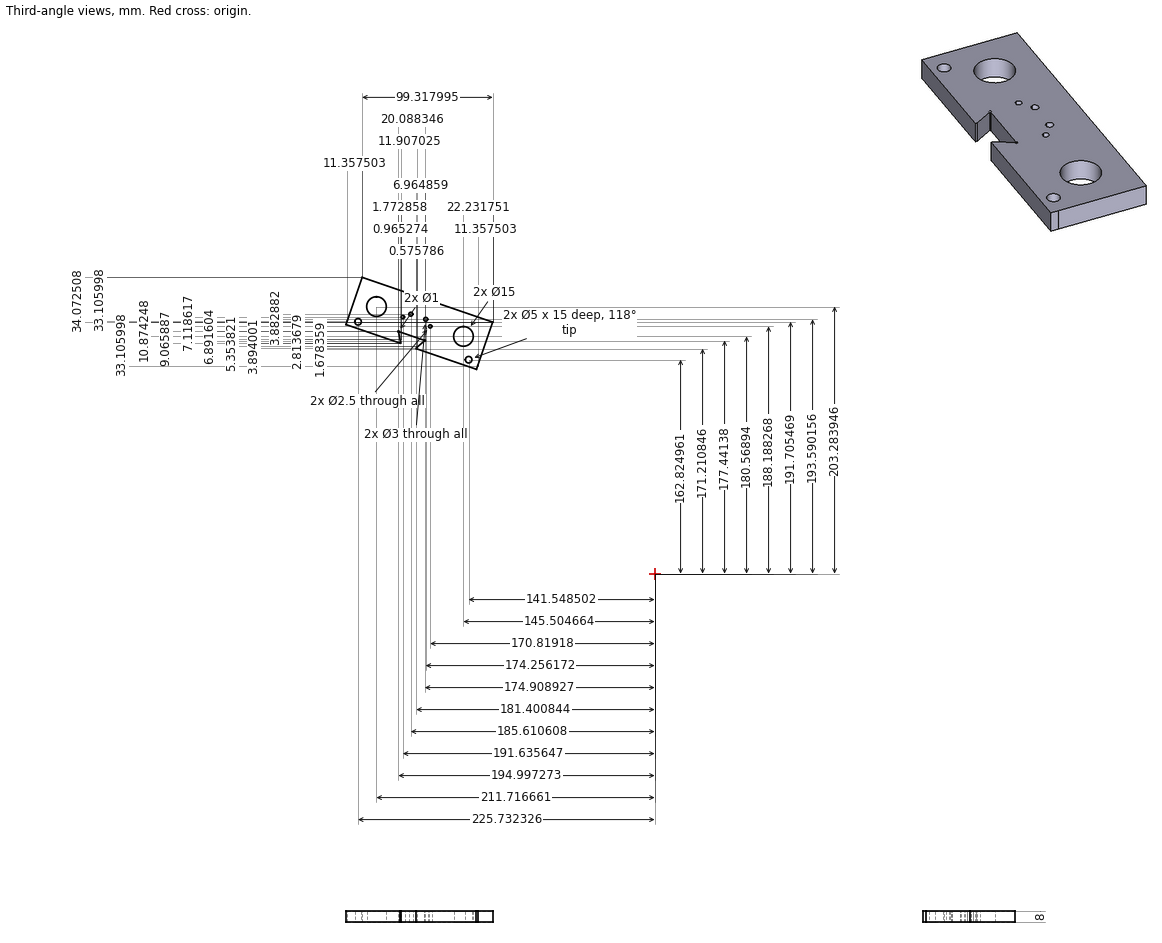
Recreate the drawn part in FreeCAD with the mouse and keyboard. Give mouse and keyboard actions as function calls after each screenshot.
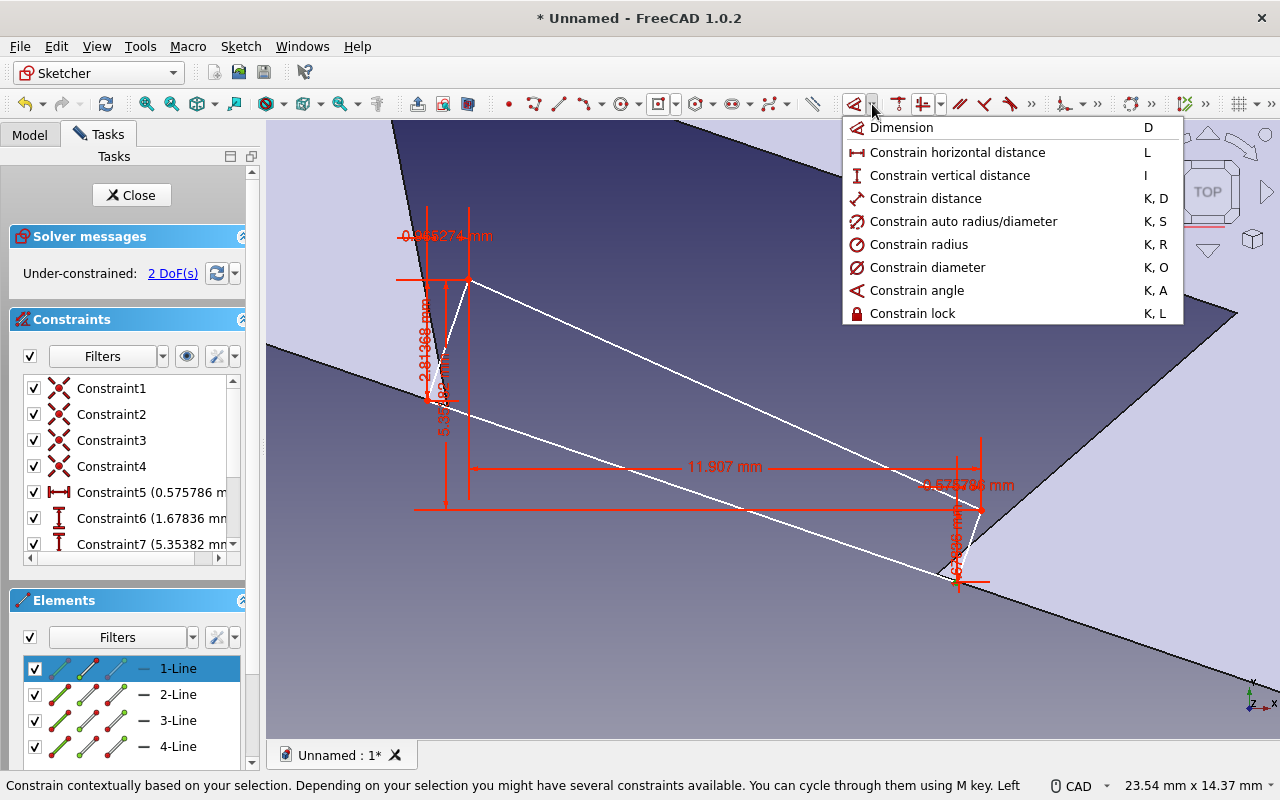
click(1013, 152)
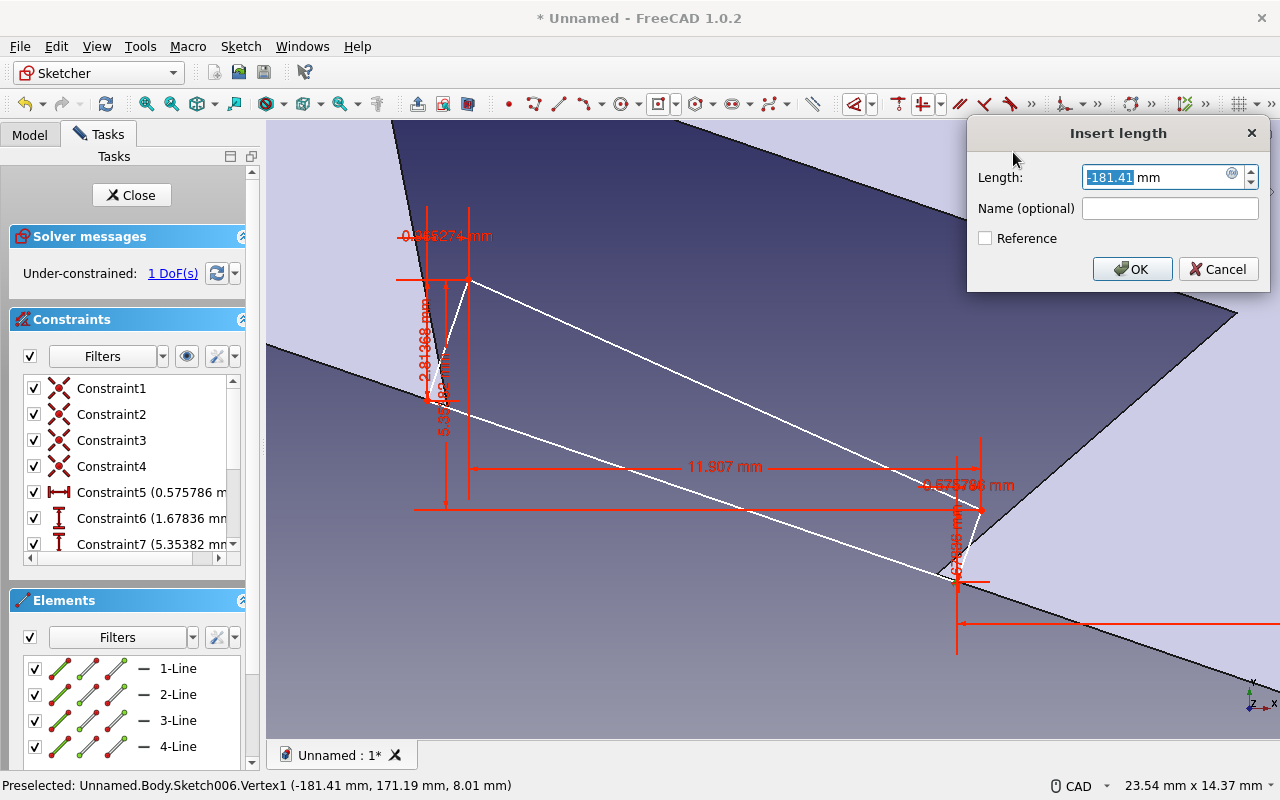
text(-181.400844)
key(Return)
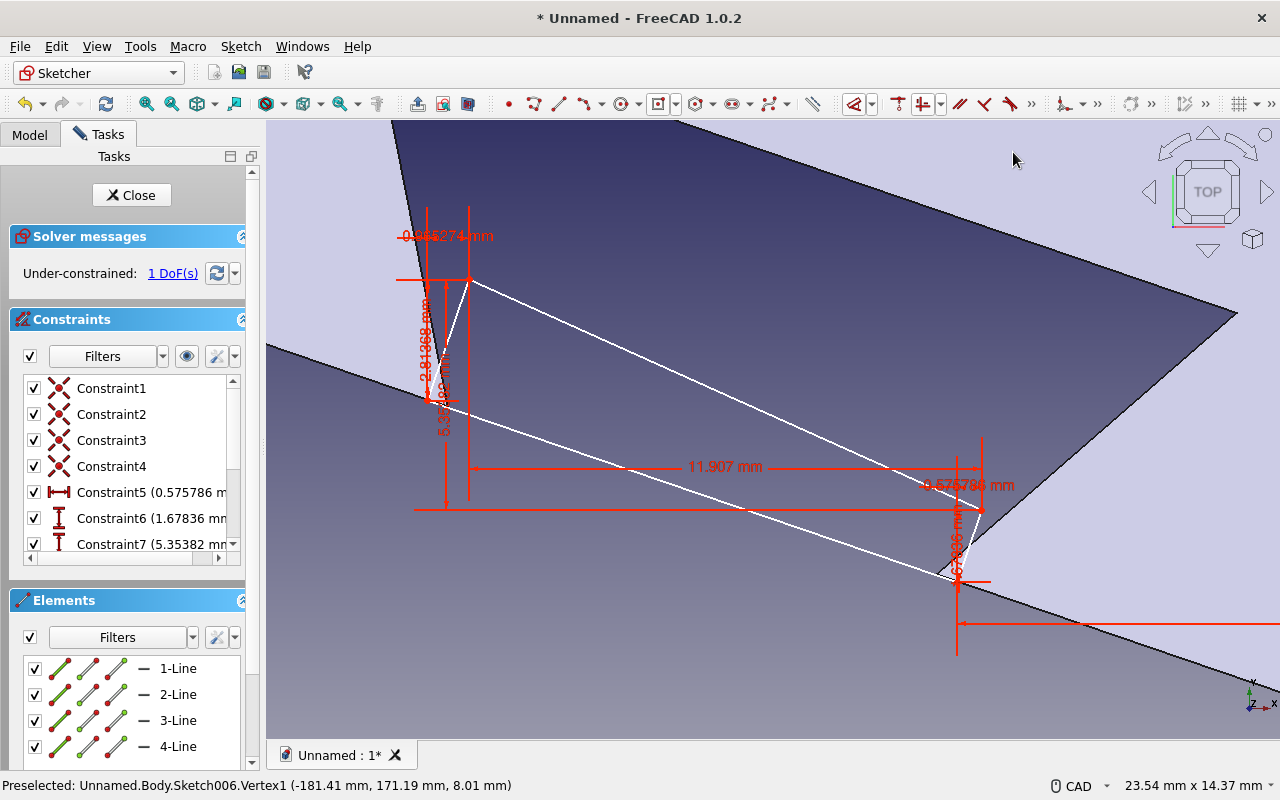
click(957, 582)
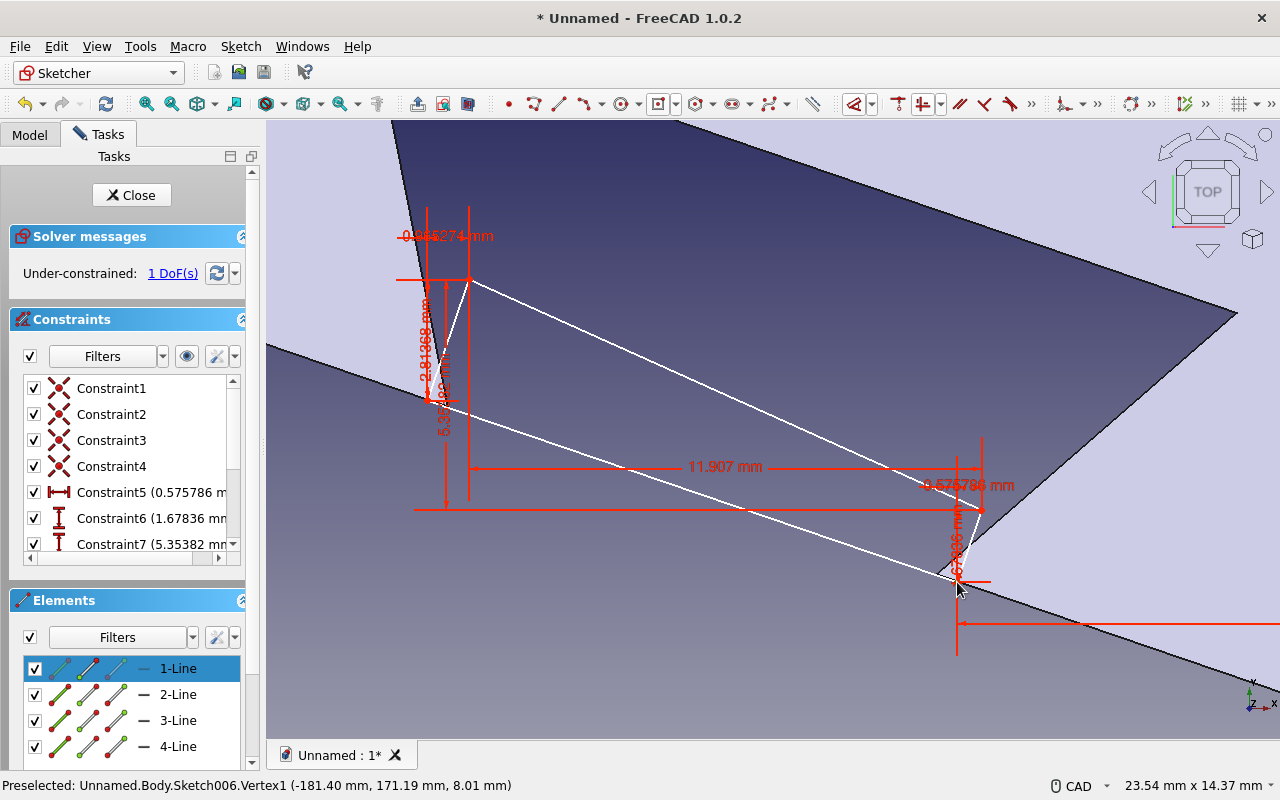
click(872, 104)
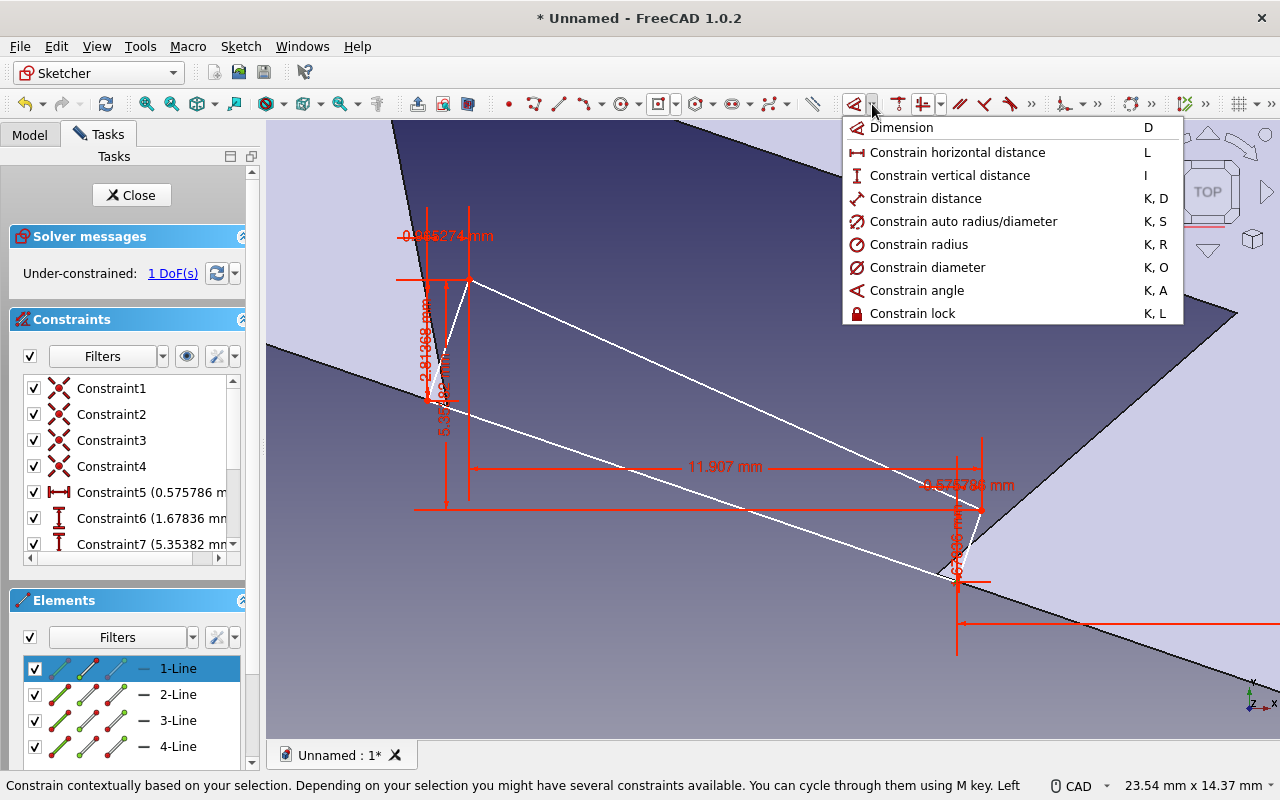
click(1013, 176)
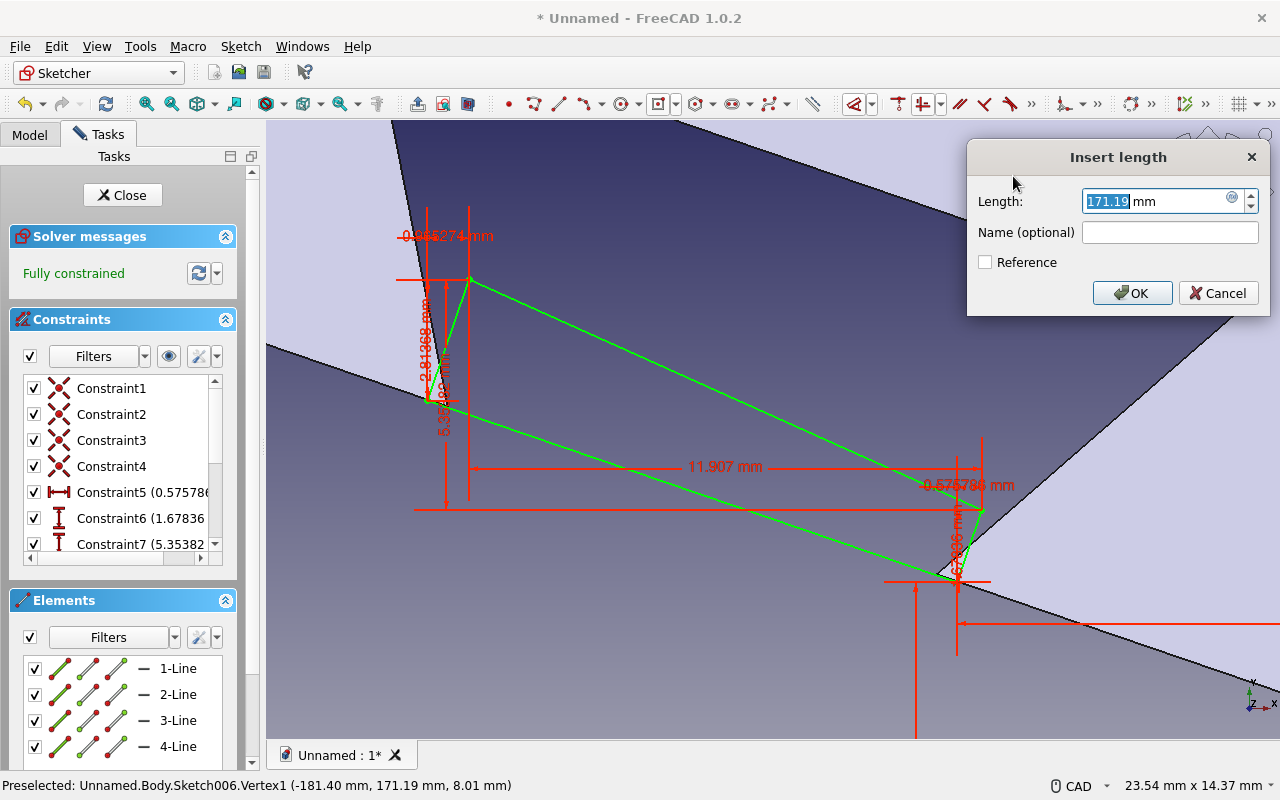
text(171.210846)
key(Return)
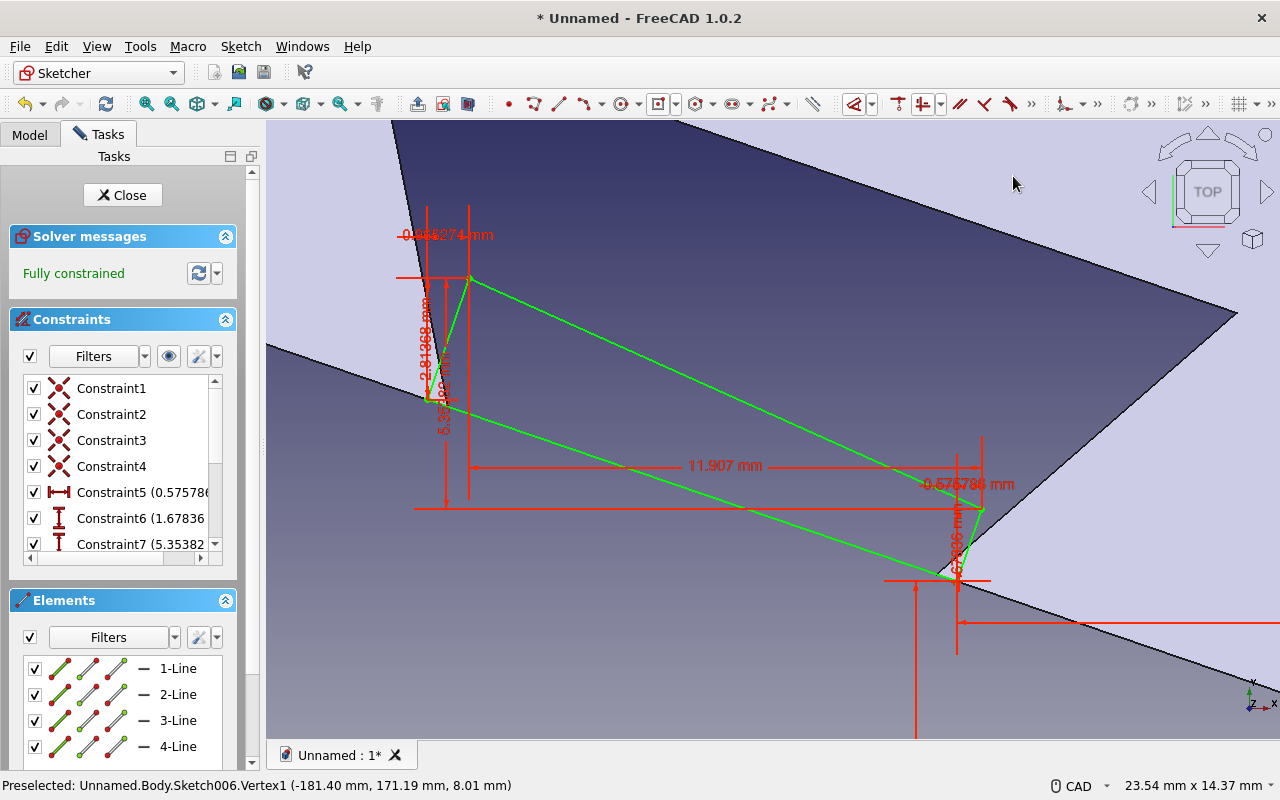
click(123, 195)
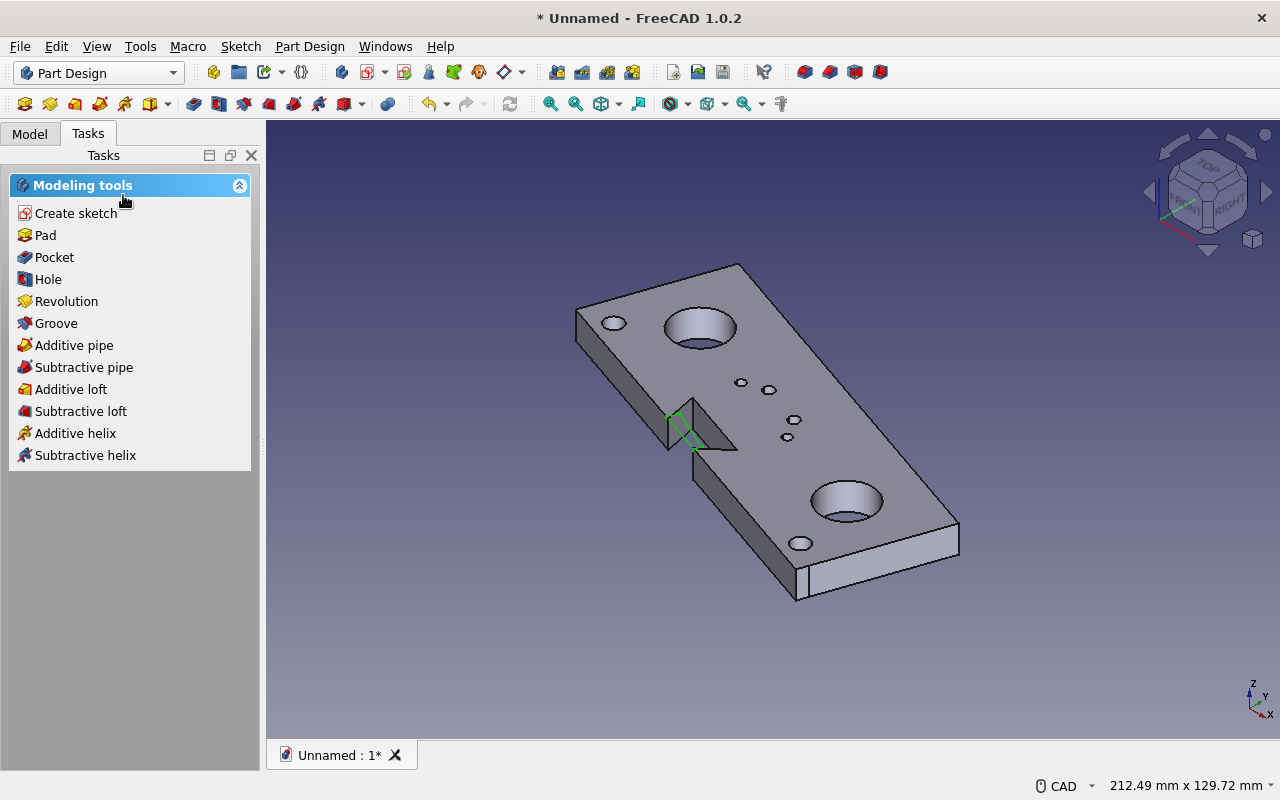
click(194, 104)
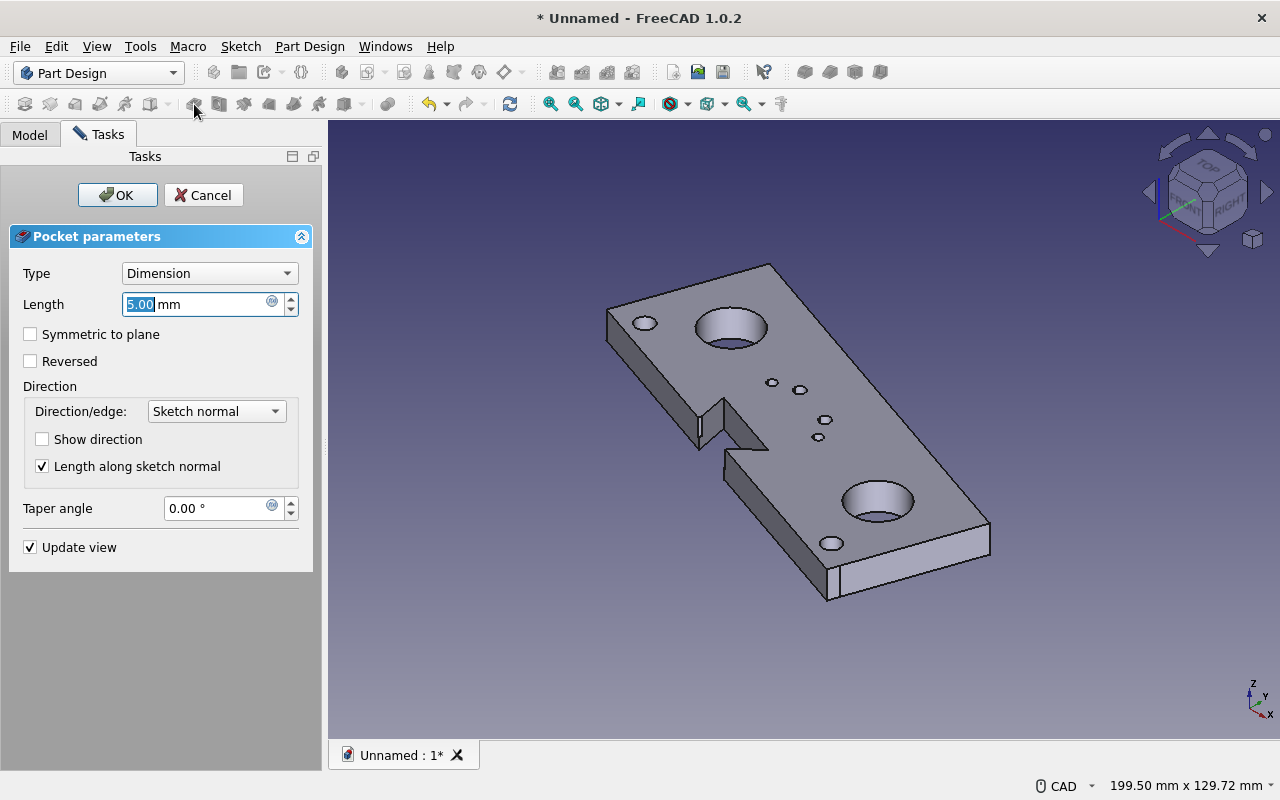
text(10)
key(Tab)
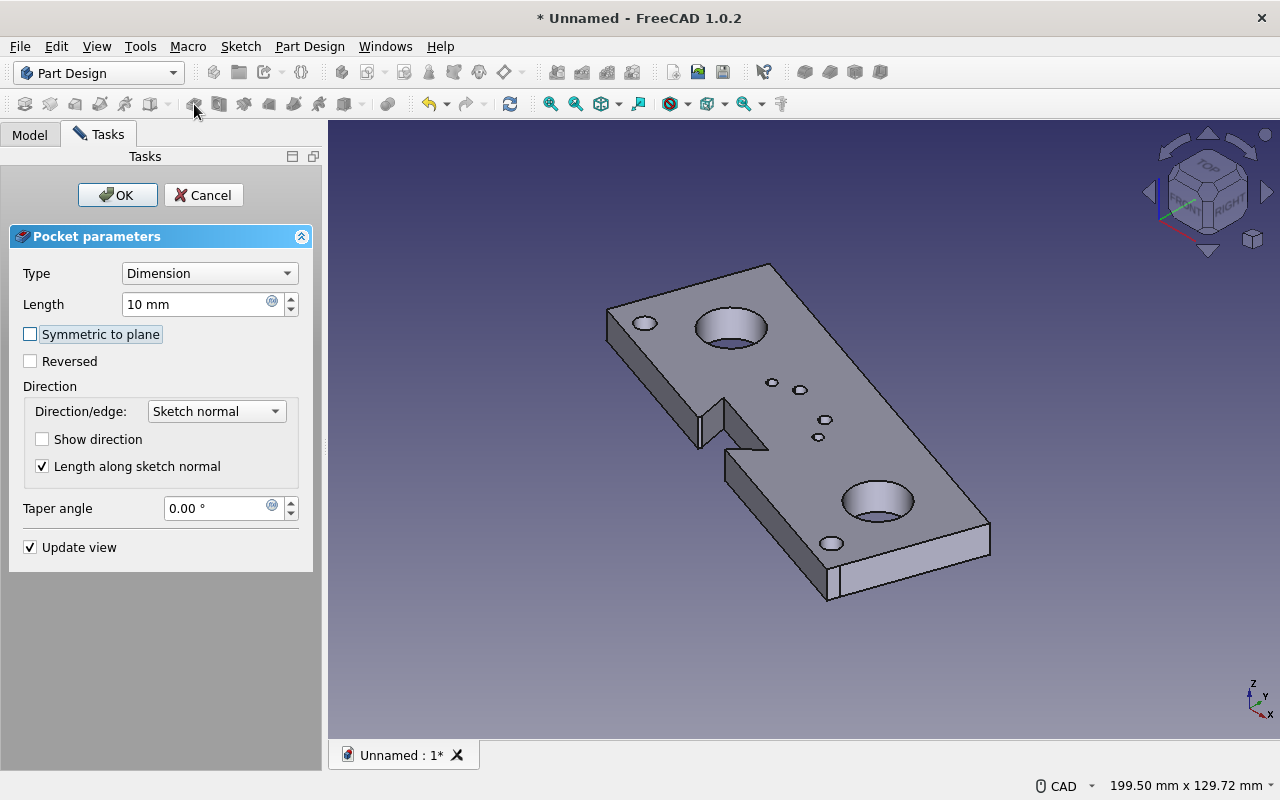
click(118, 195)